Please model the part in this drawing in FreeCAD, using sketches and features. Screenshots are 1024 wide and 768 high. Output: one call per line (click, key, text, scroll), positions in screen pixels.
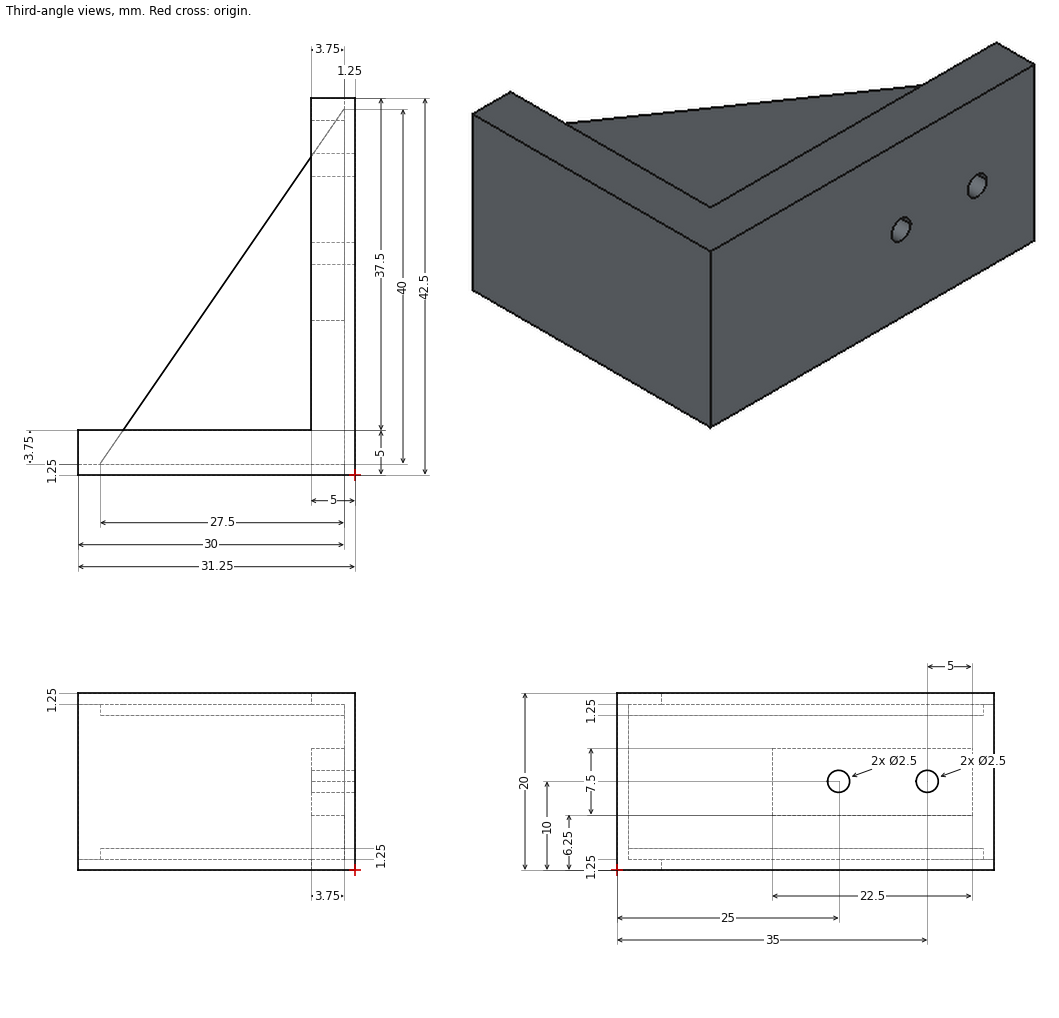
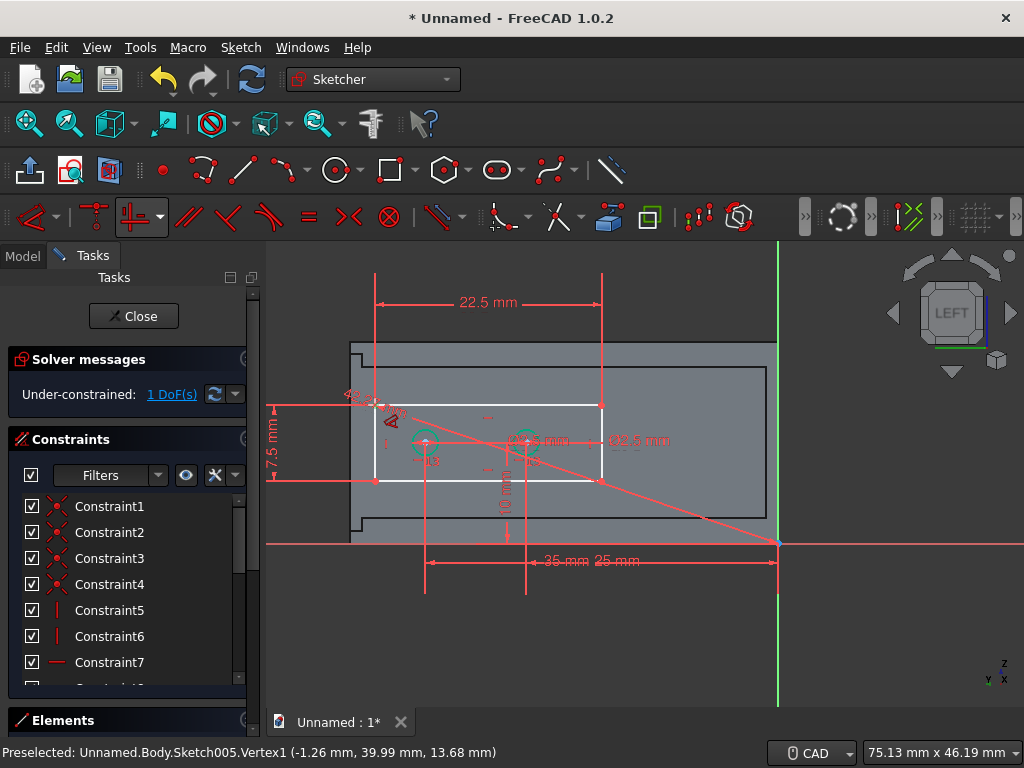
click(425, 443)
click(400, 371)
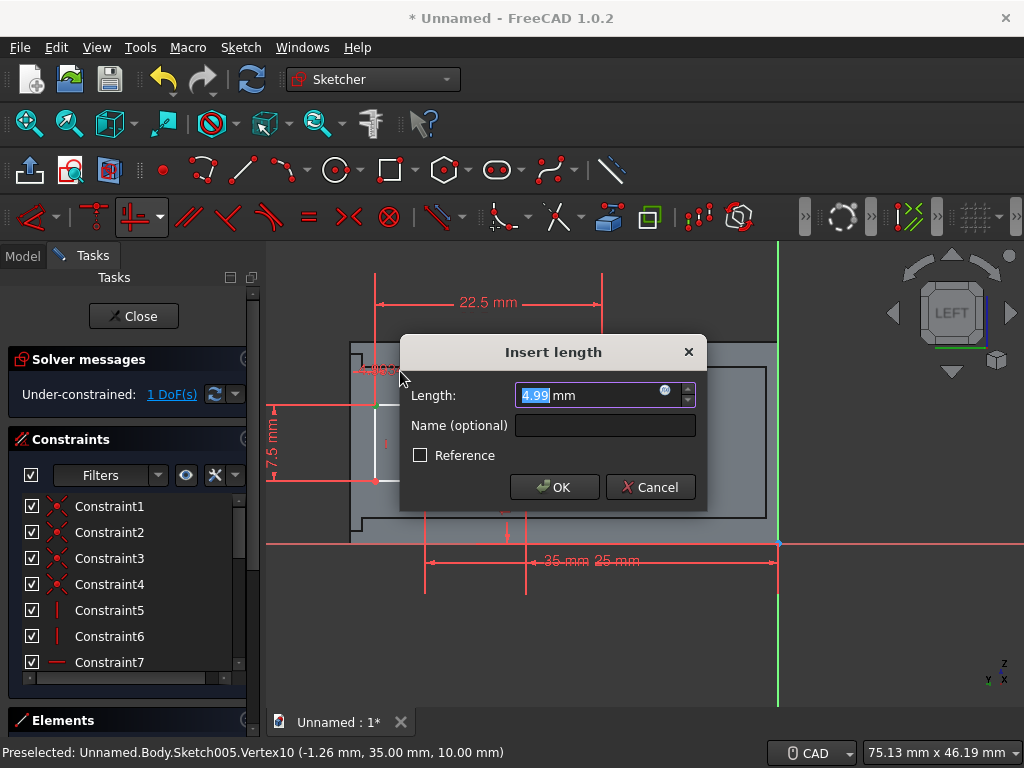
text(5)
key(Return)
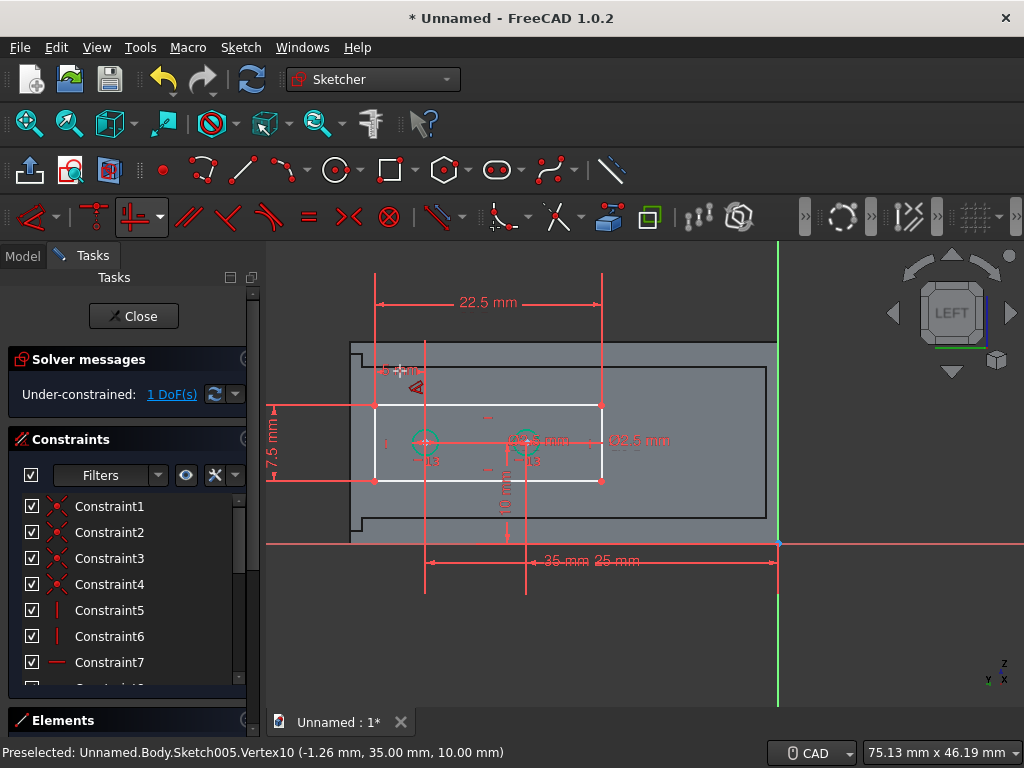
click(375, 481)
click(812, 512)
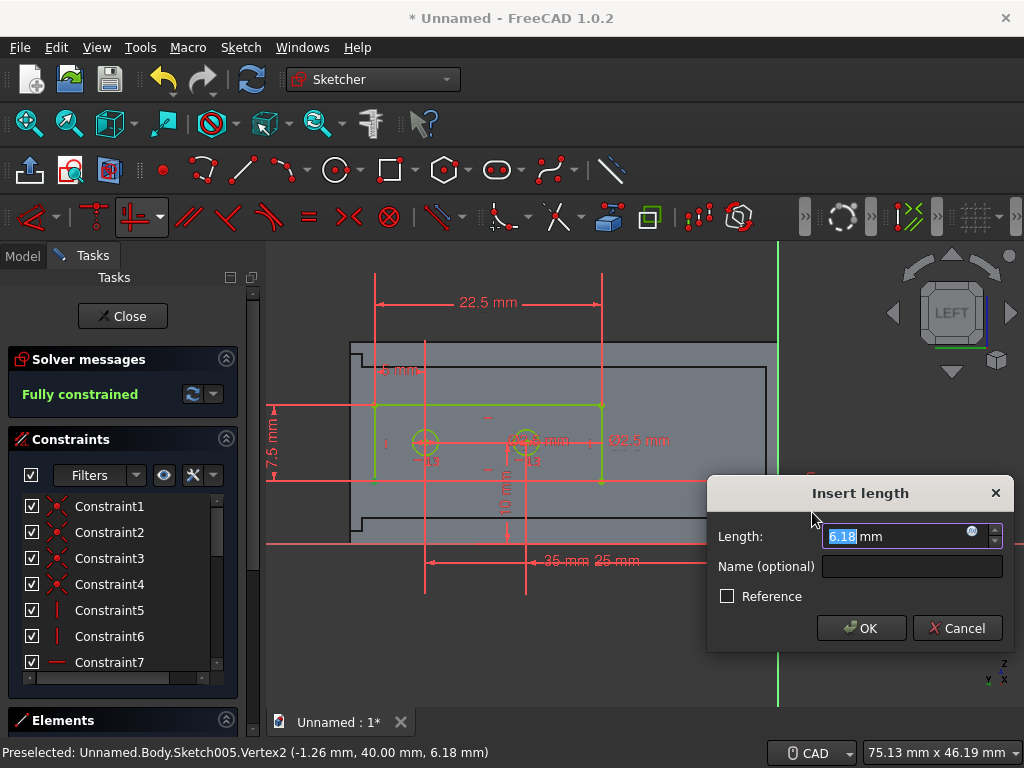
text(6.25)
key(Return)
key(Escape)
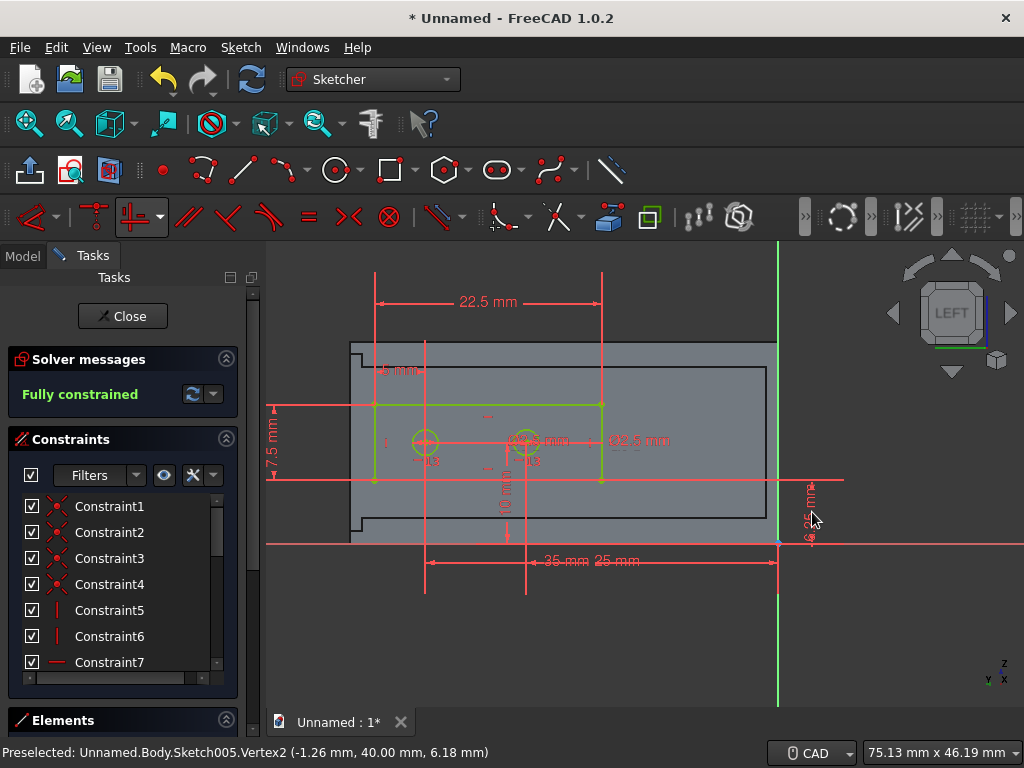
click(123, 316)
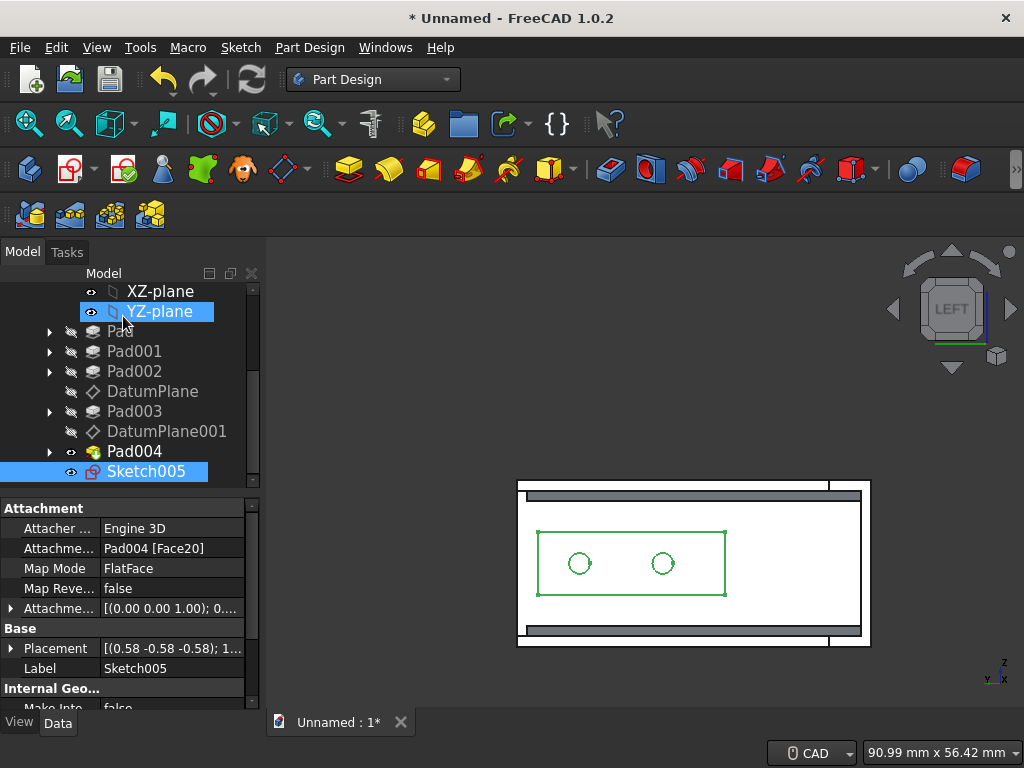
click(350, 170)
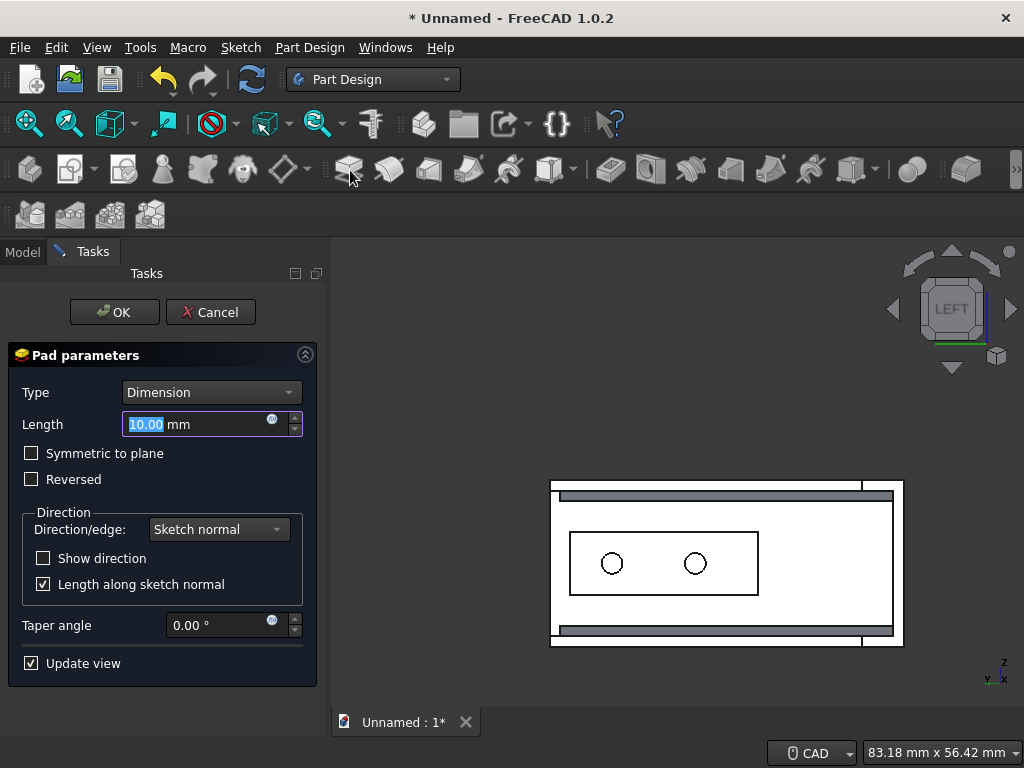
text(3.75)
key(Tab)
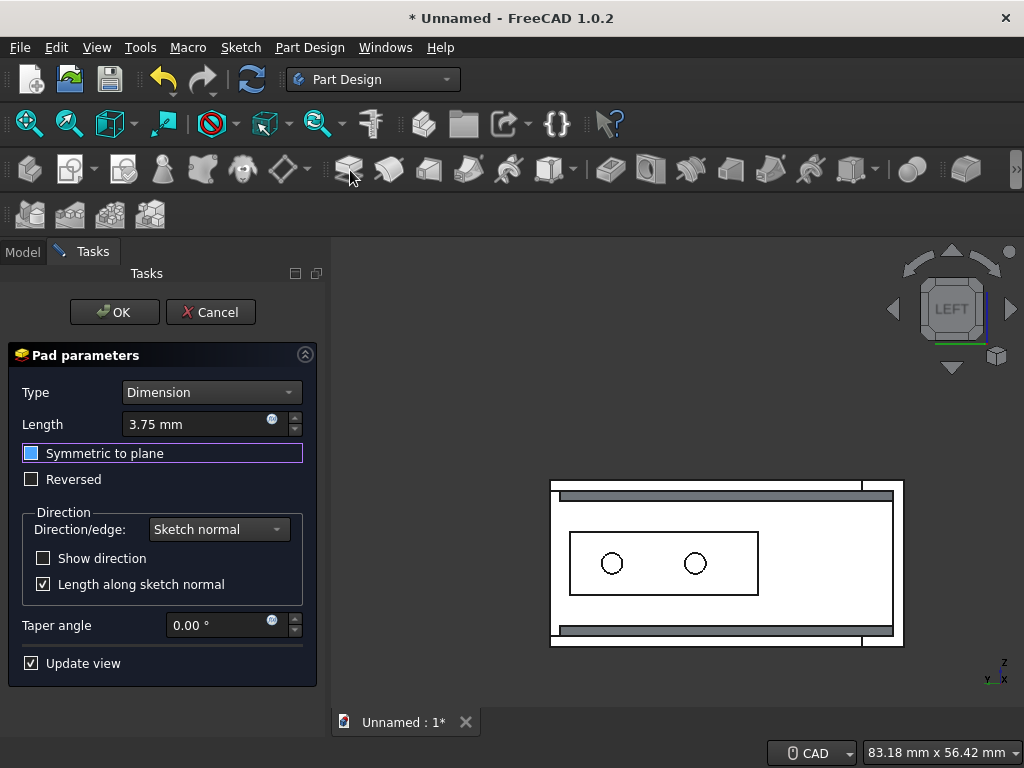
click(115, 312)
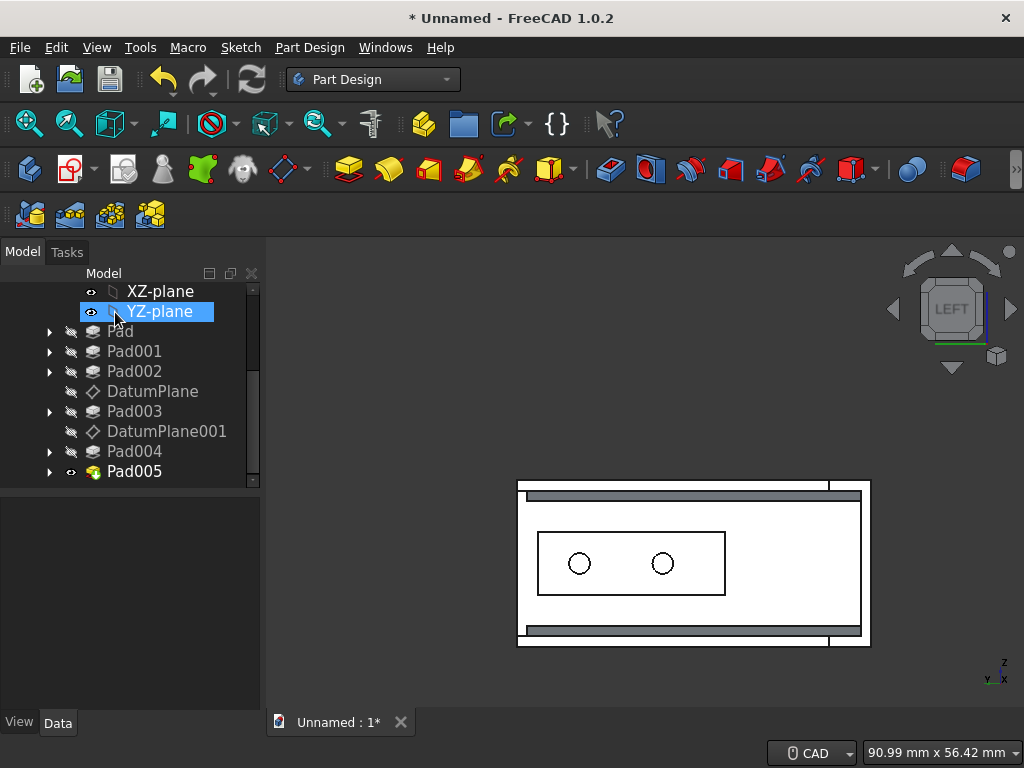
scroll(160, 387, down, 3)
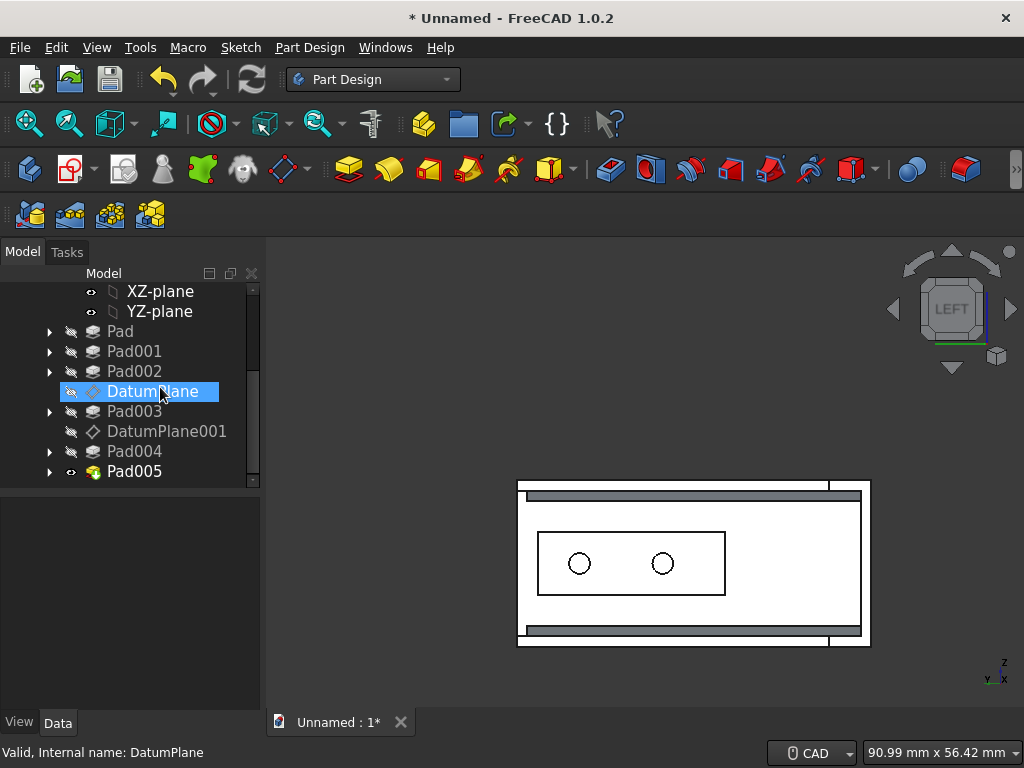
scroll(160, 387, up, 15)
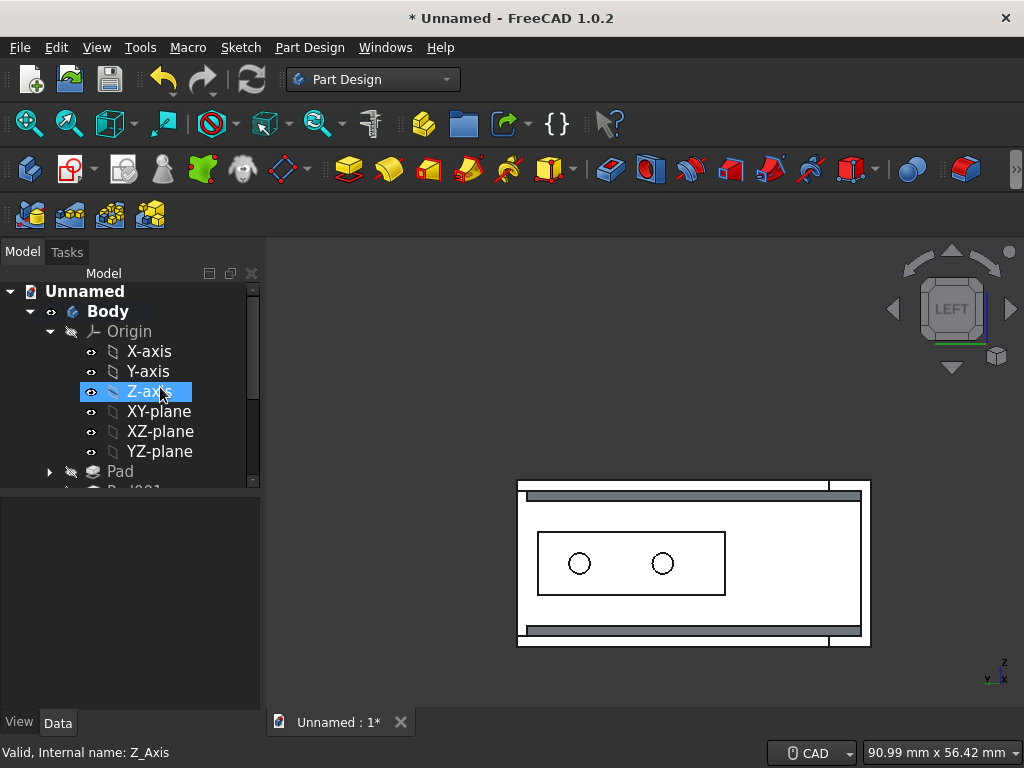
click(136, 452)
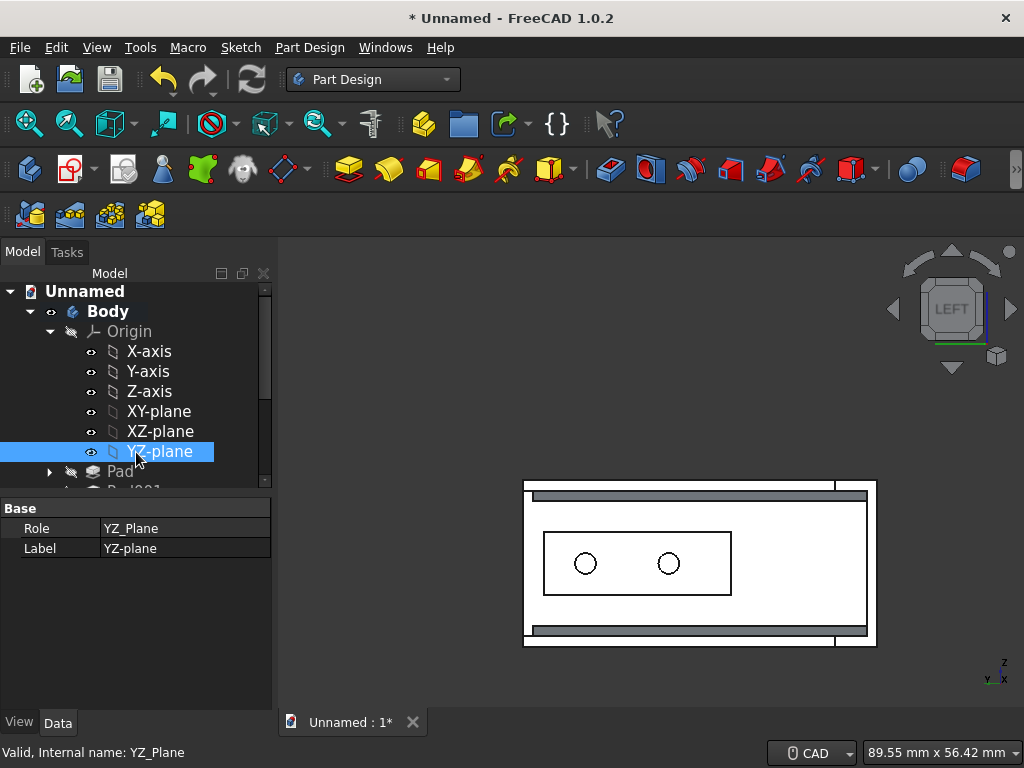
click(284, 170)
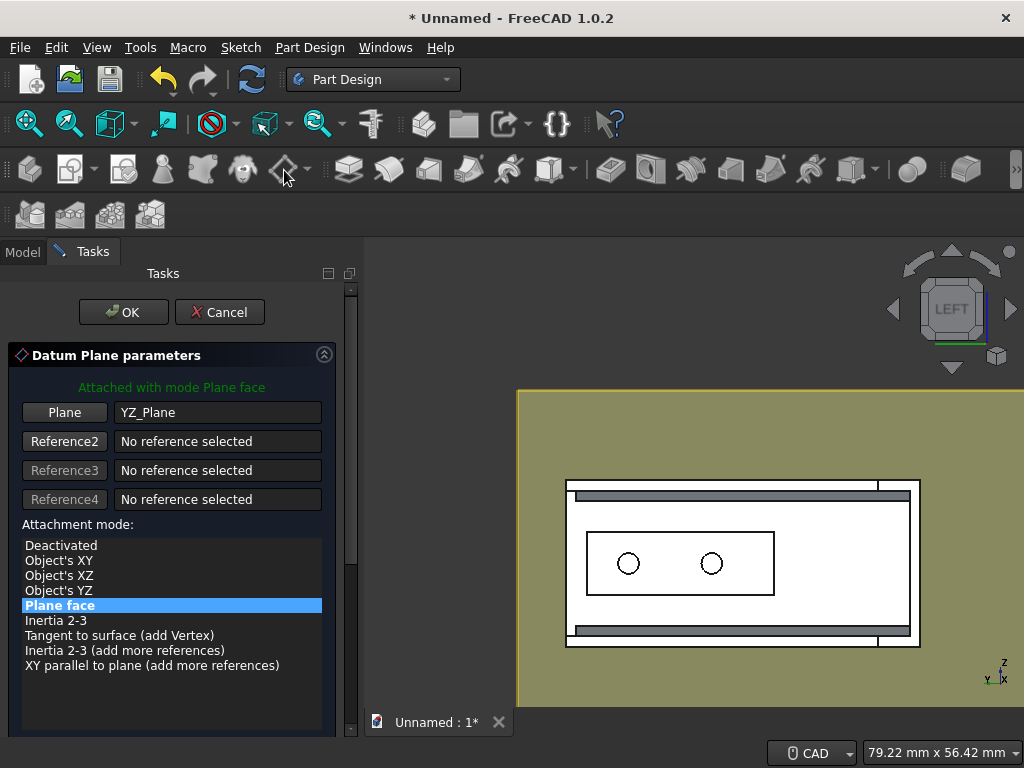
scroll(351, 510, down, 3)